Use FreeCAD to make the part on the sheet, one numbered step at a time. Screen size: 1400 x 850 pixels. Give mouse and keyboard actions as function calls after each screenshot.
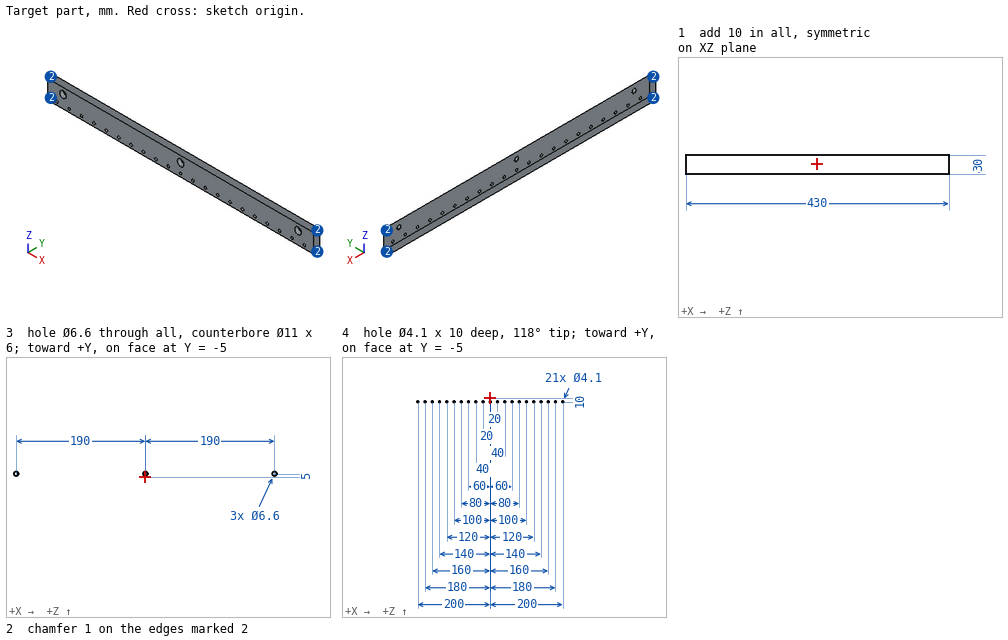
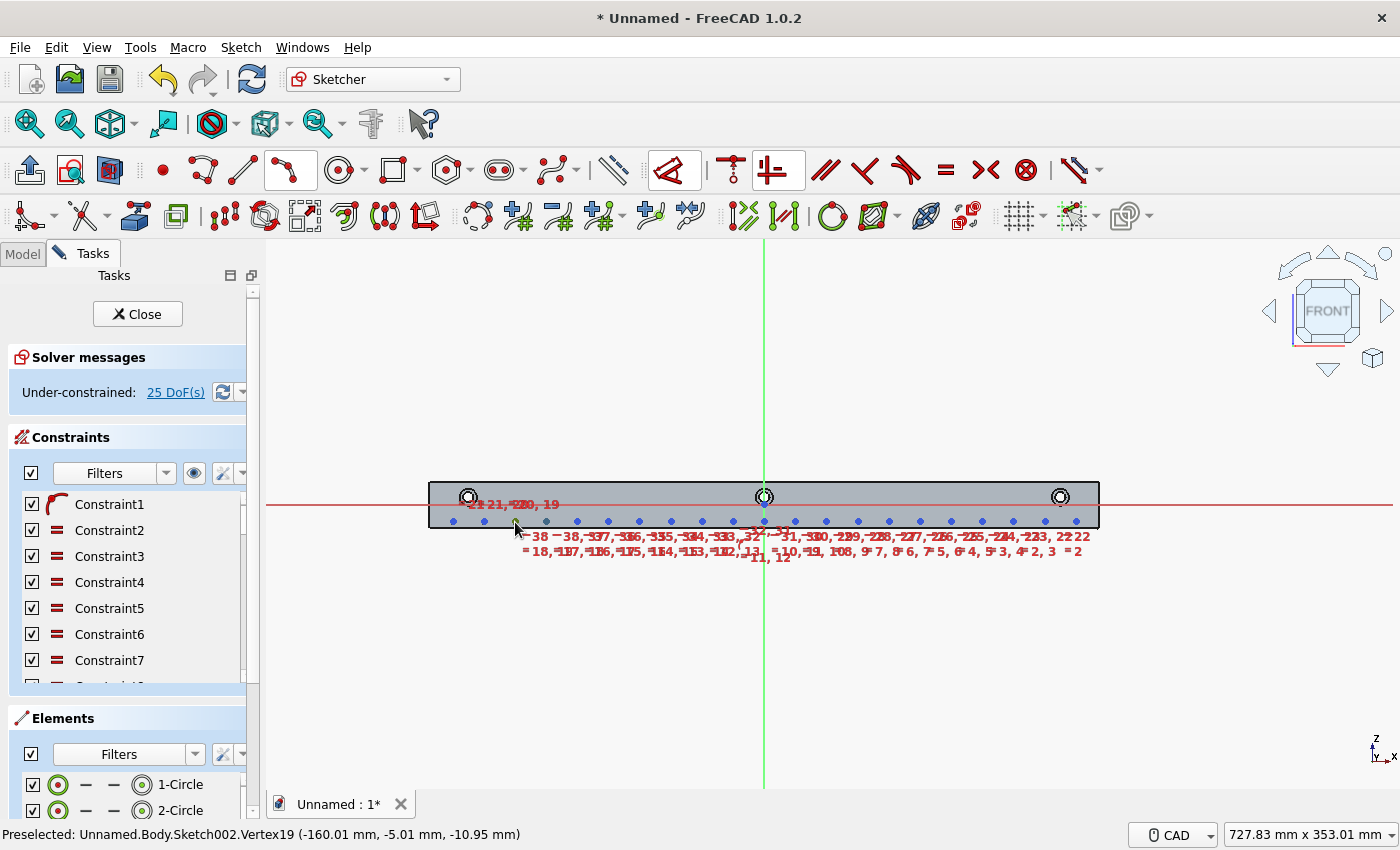
key(h)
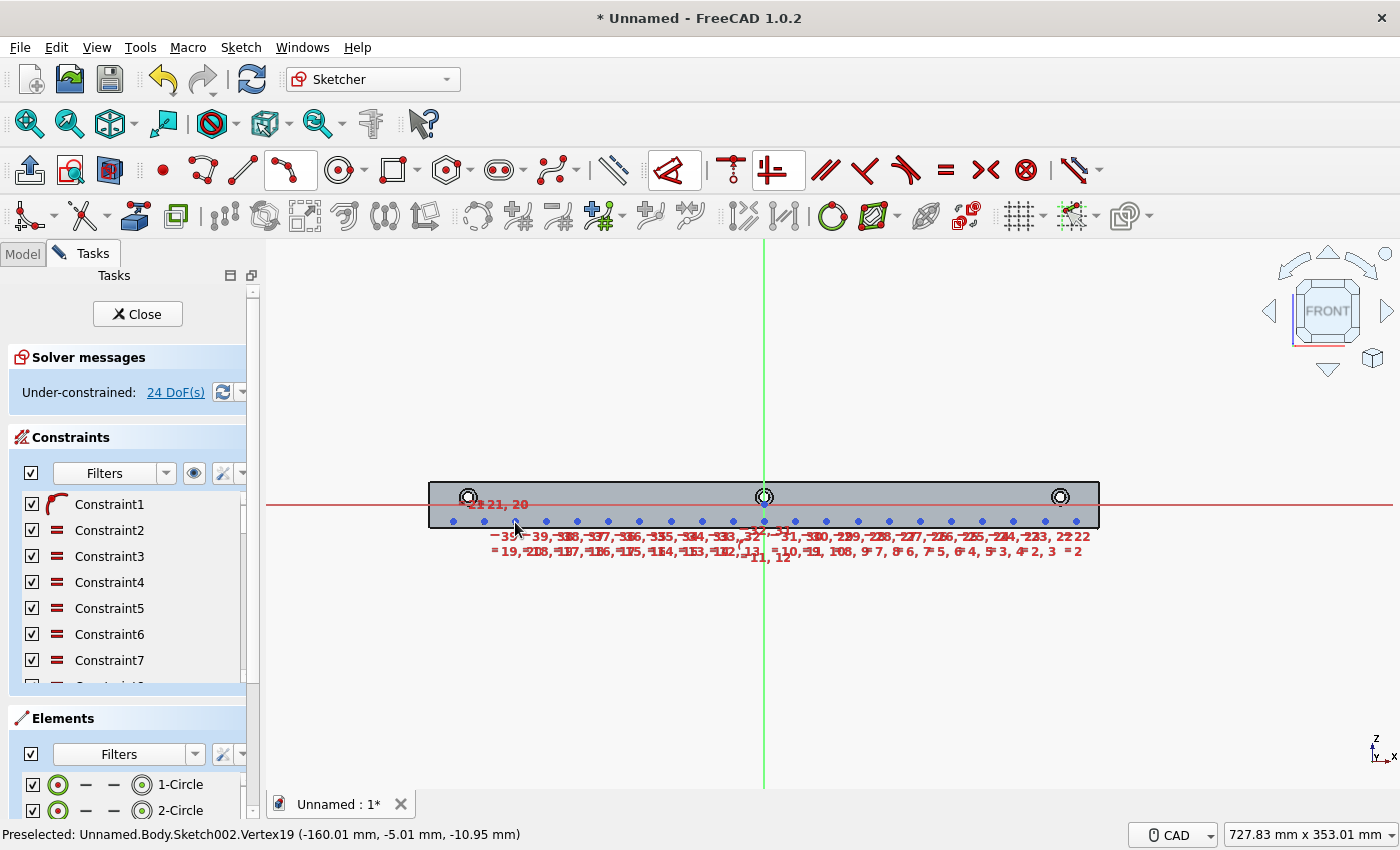
click(515, 522)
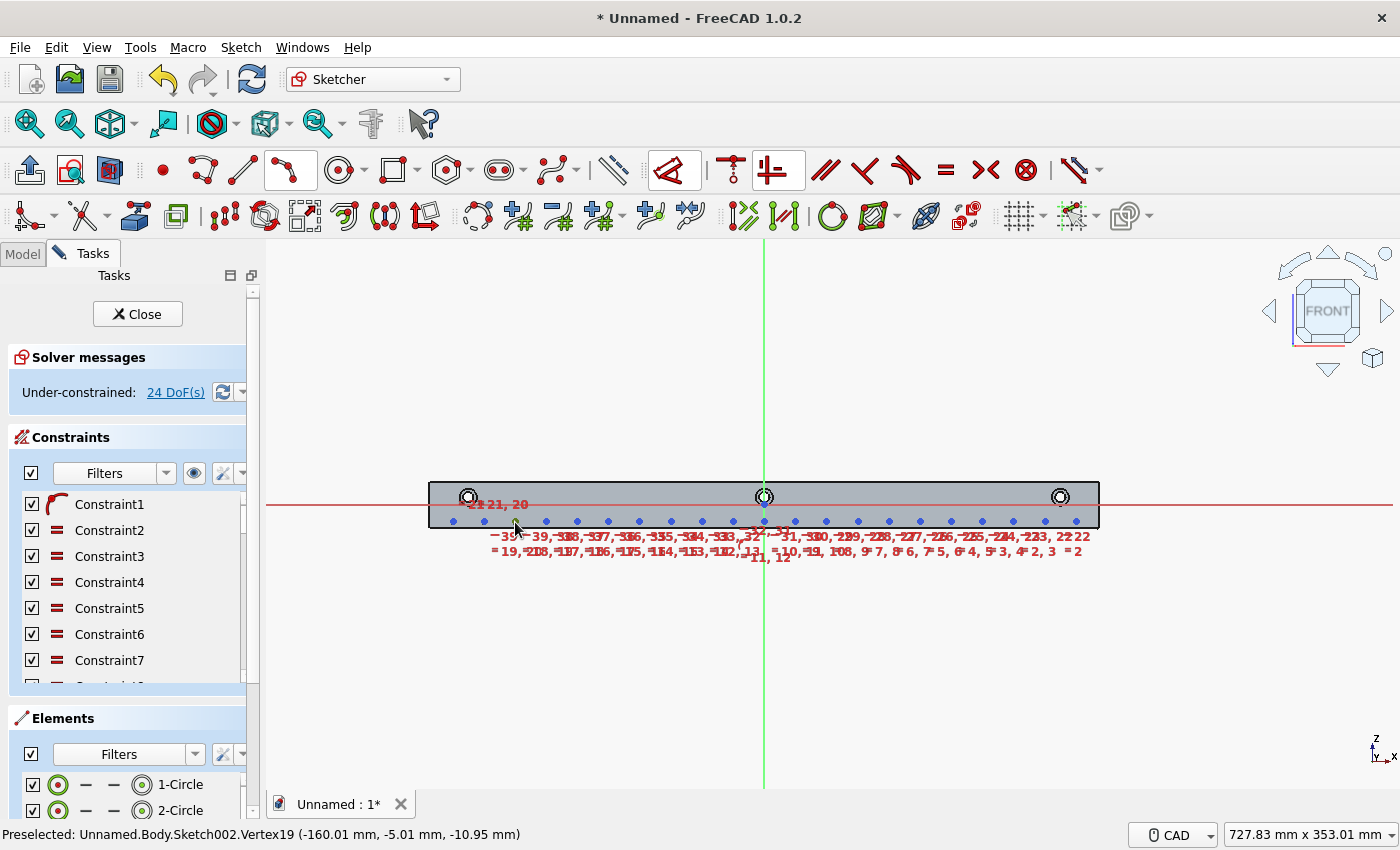
click(484, 522)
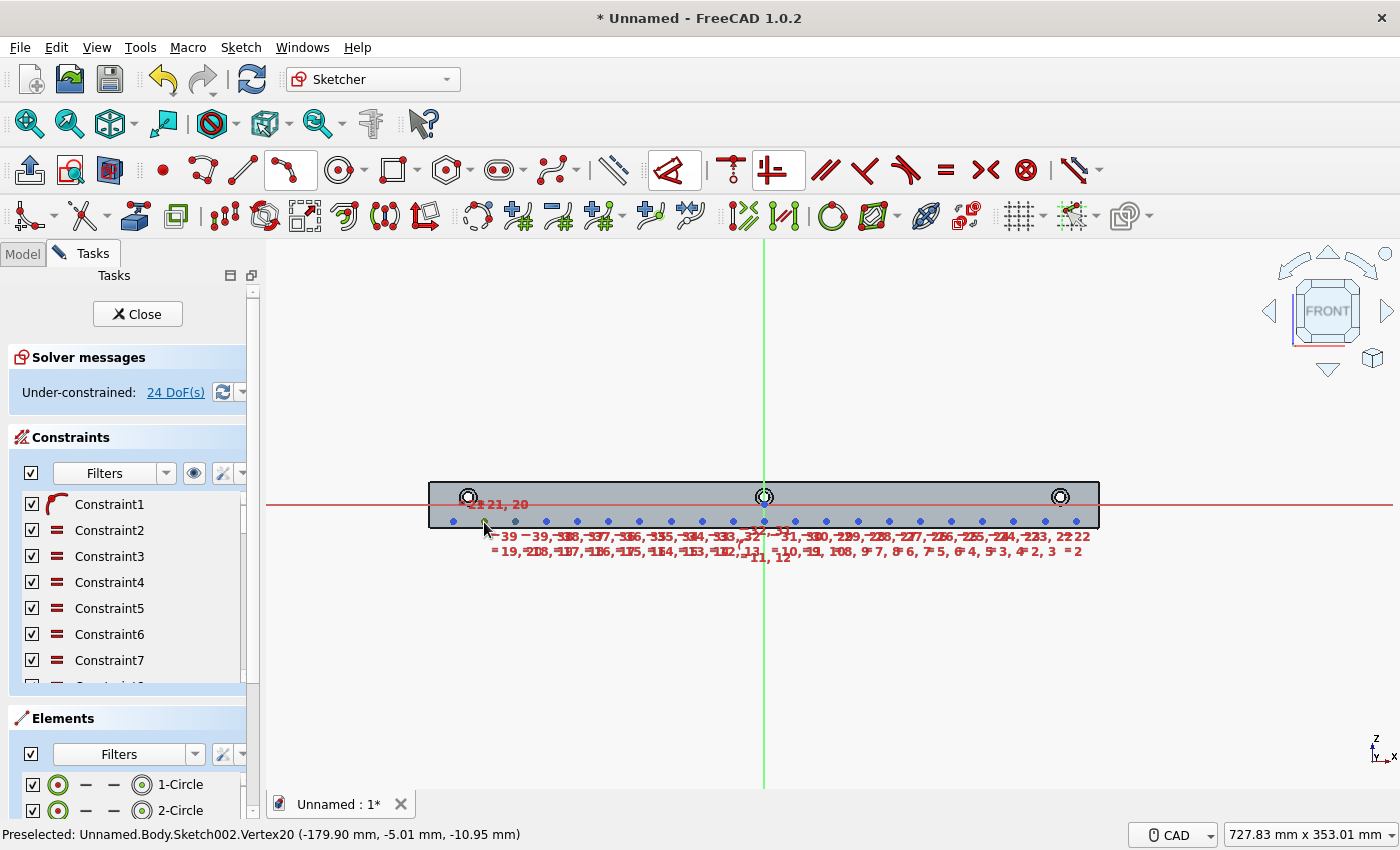
click(800, 170)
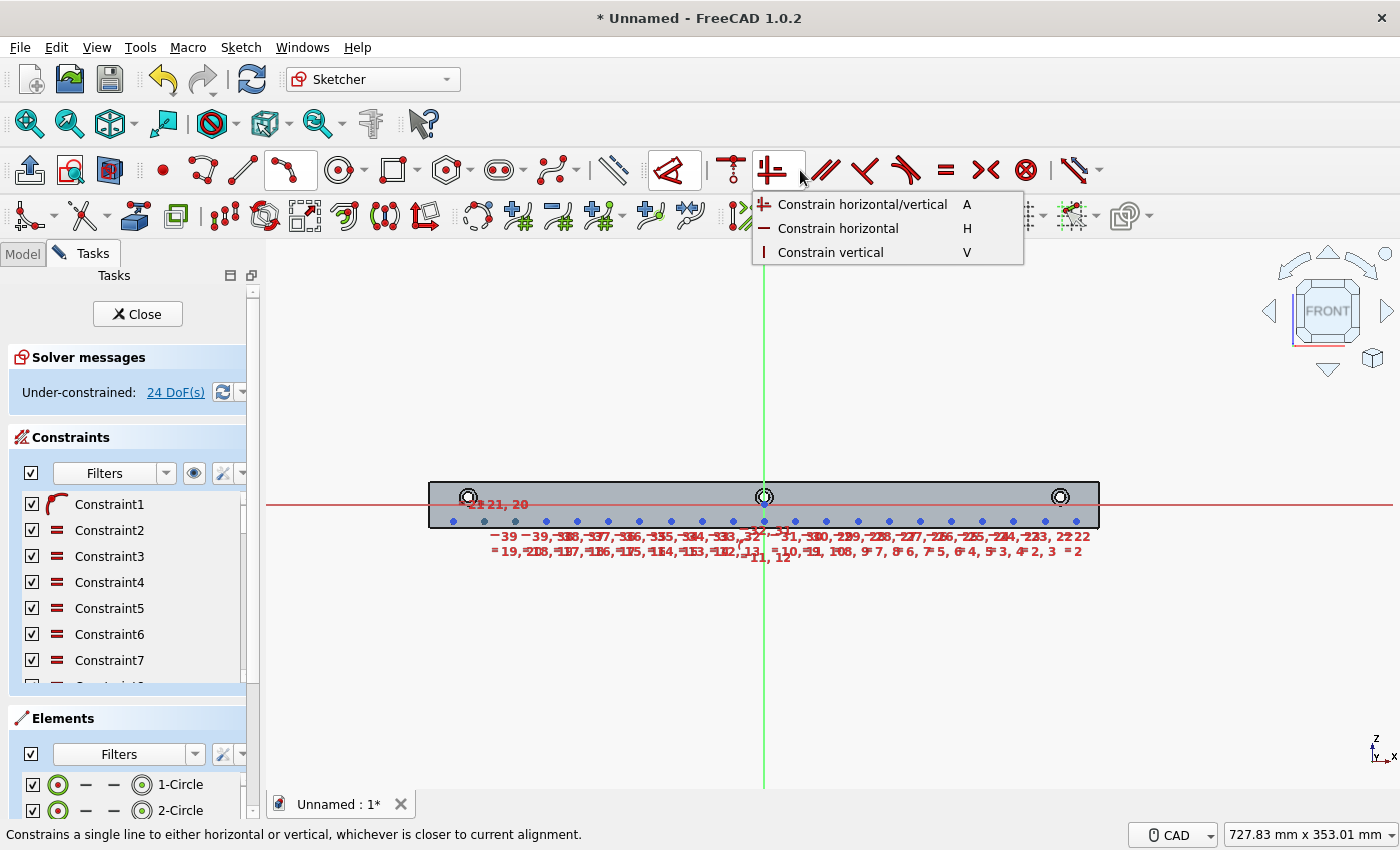
click(888, 228)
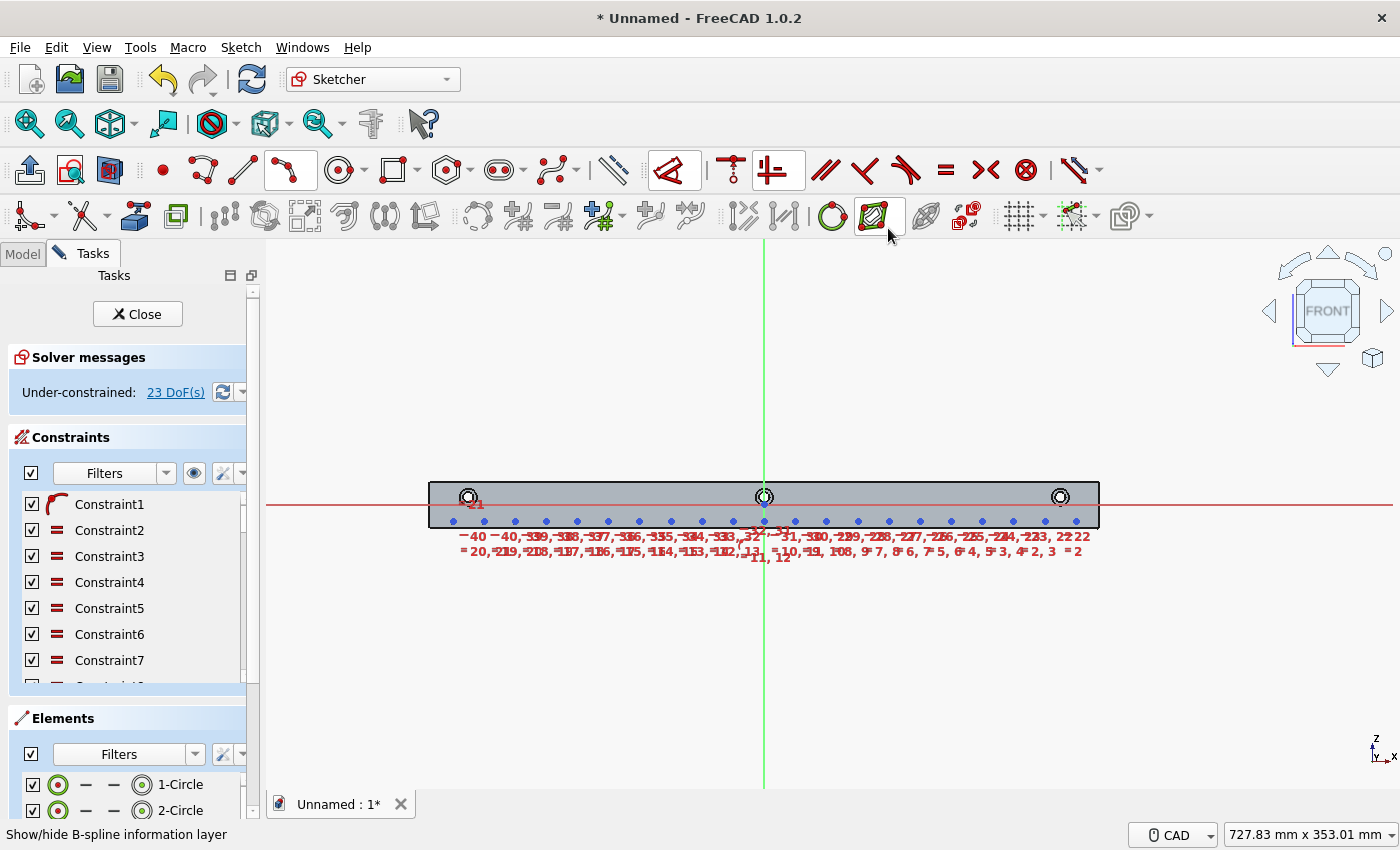
click(484, 522)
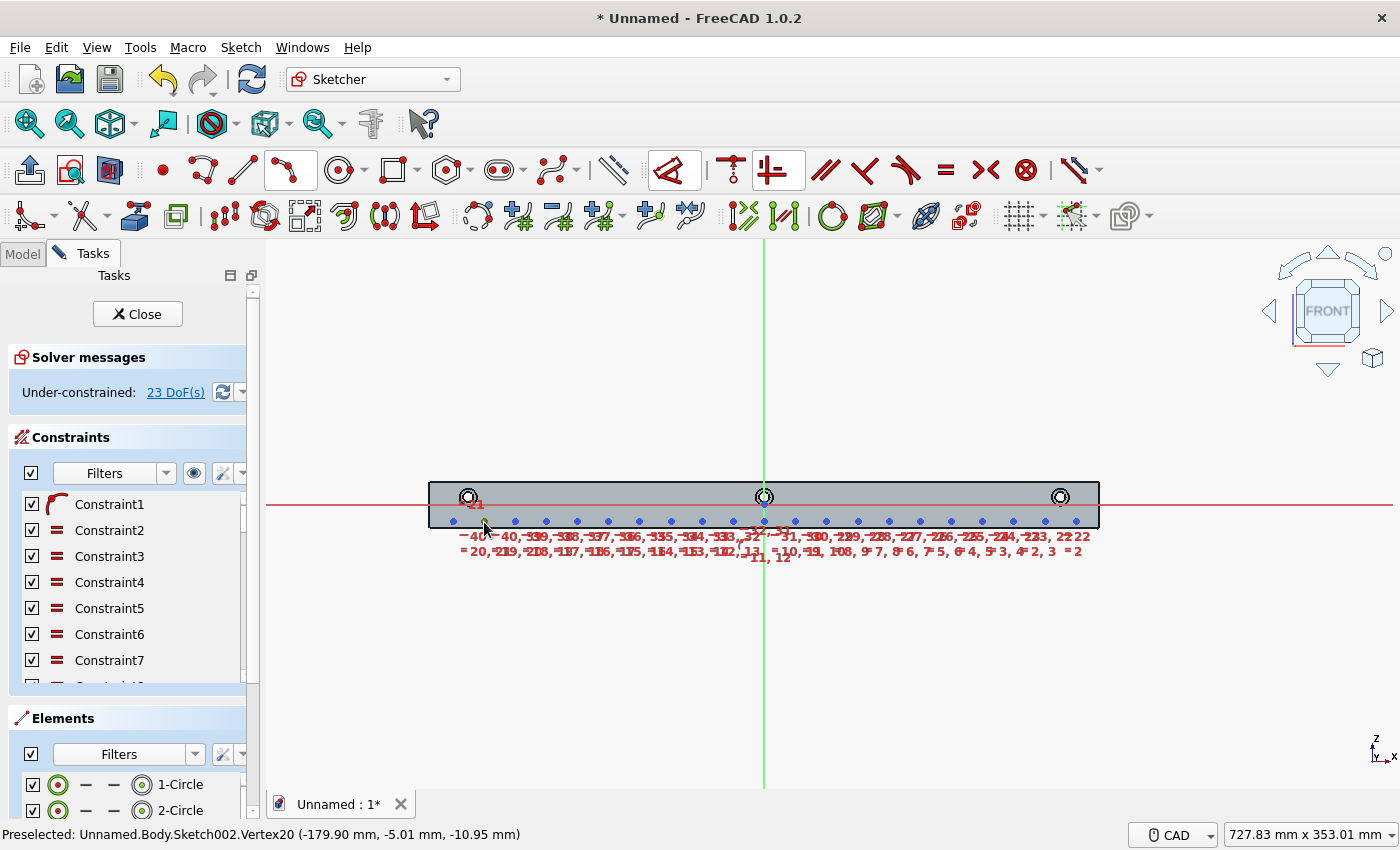
click(453, 522)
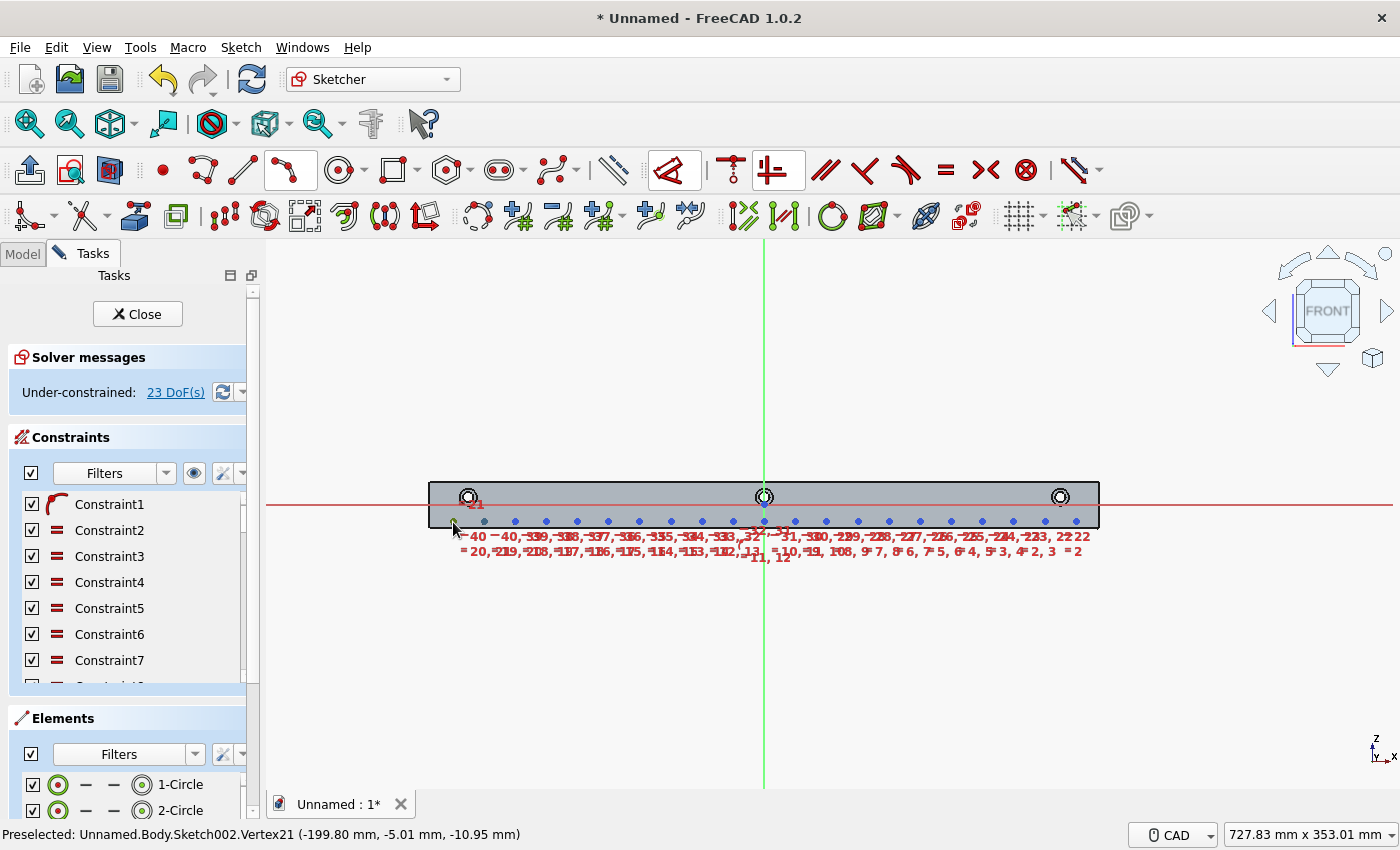
click(800, 170)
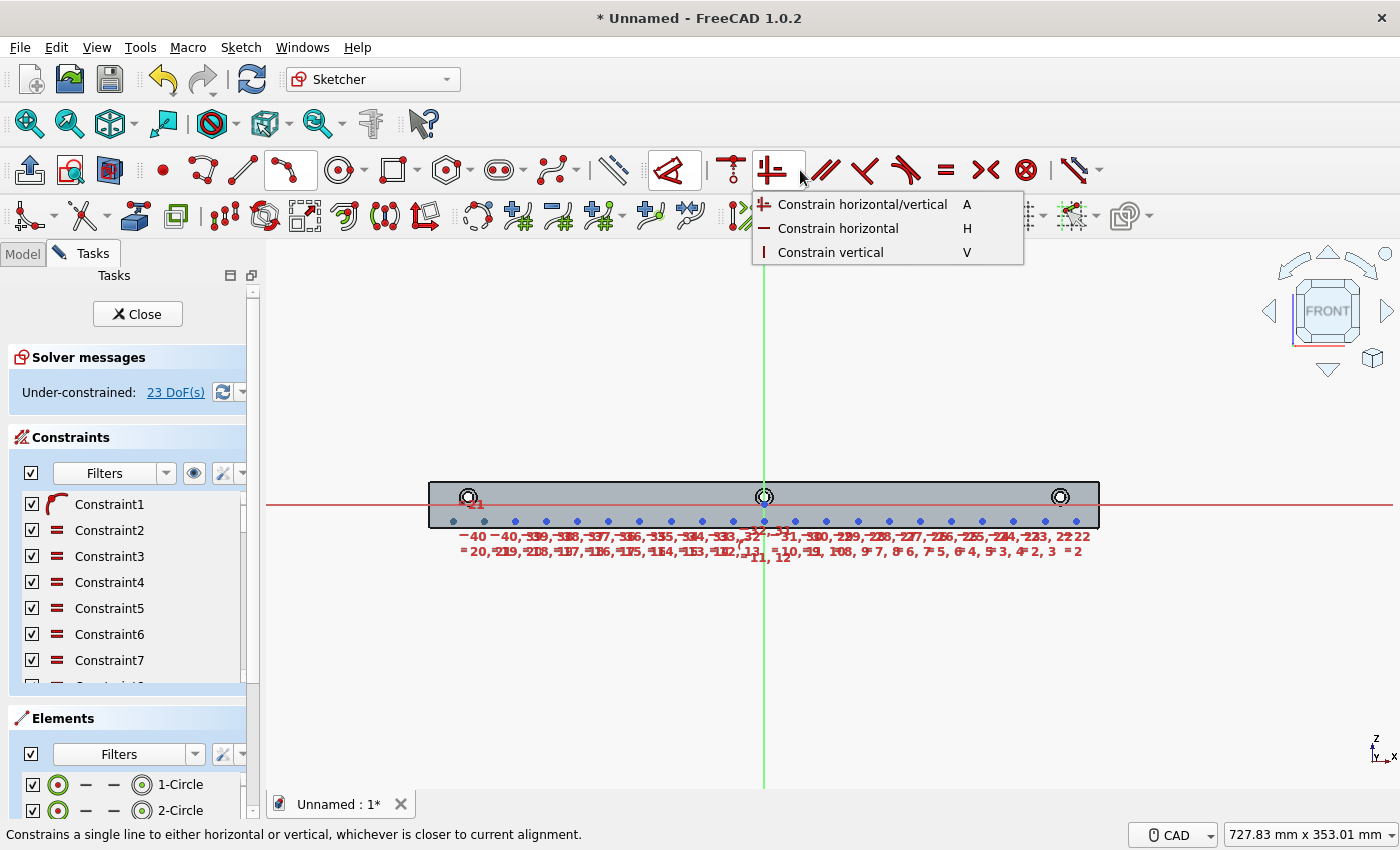
click(888, 228)